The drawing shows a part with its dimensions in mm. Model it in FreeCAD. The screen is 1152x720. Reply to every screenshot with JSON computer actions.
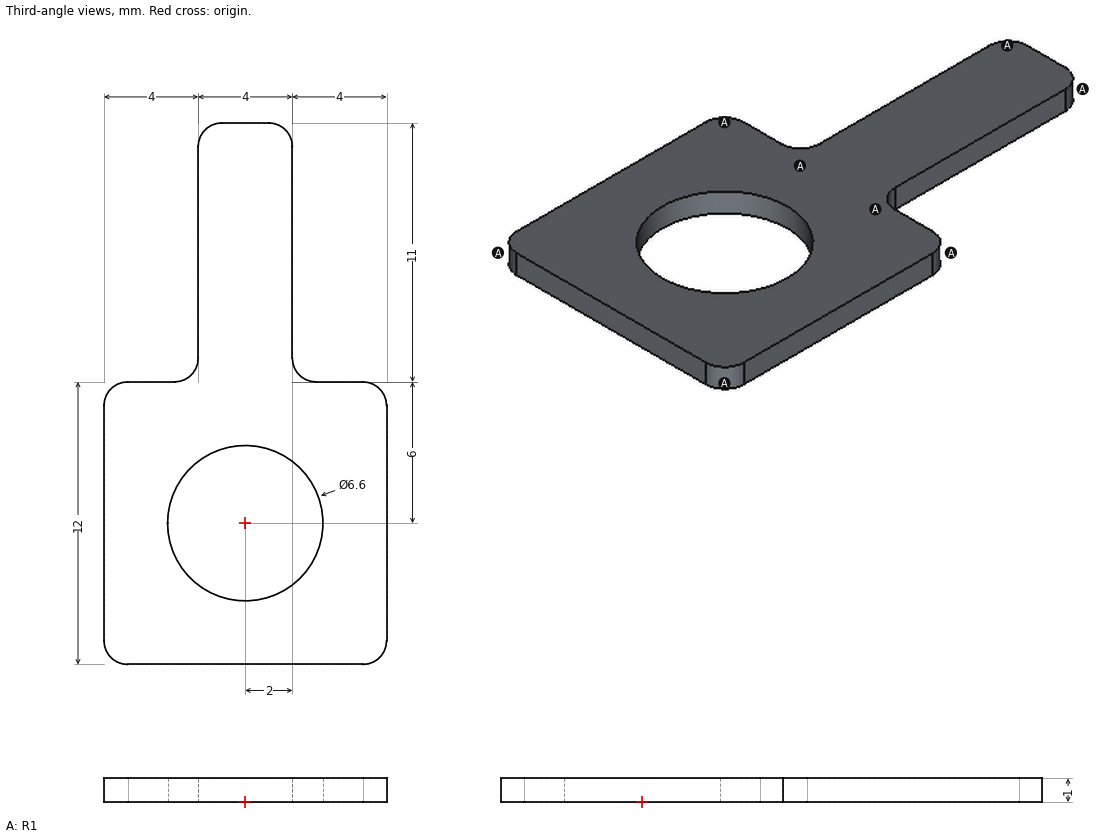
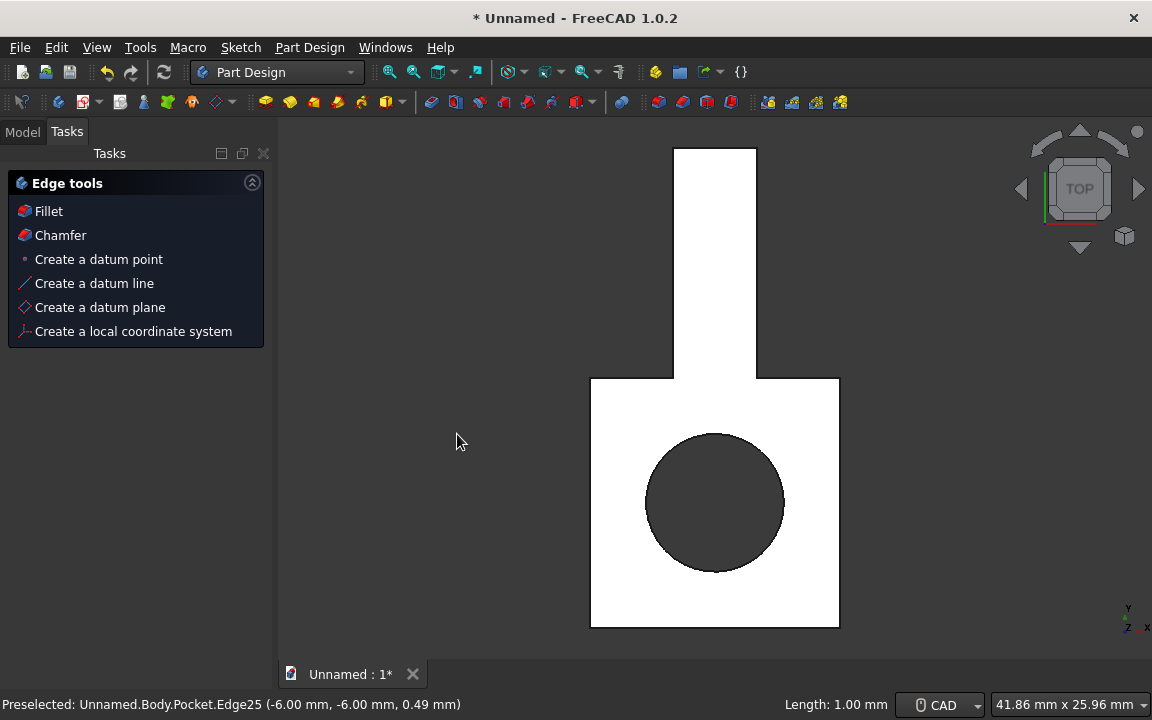
{"action": "scroll", "coordinate": [590, 627], "scroll_direction": "up", "scroll_amount": 4}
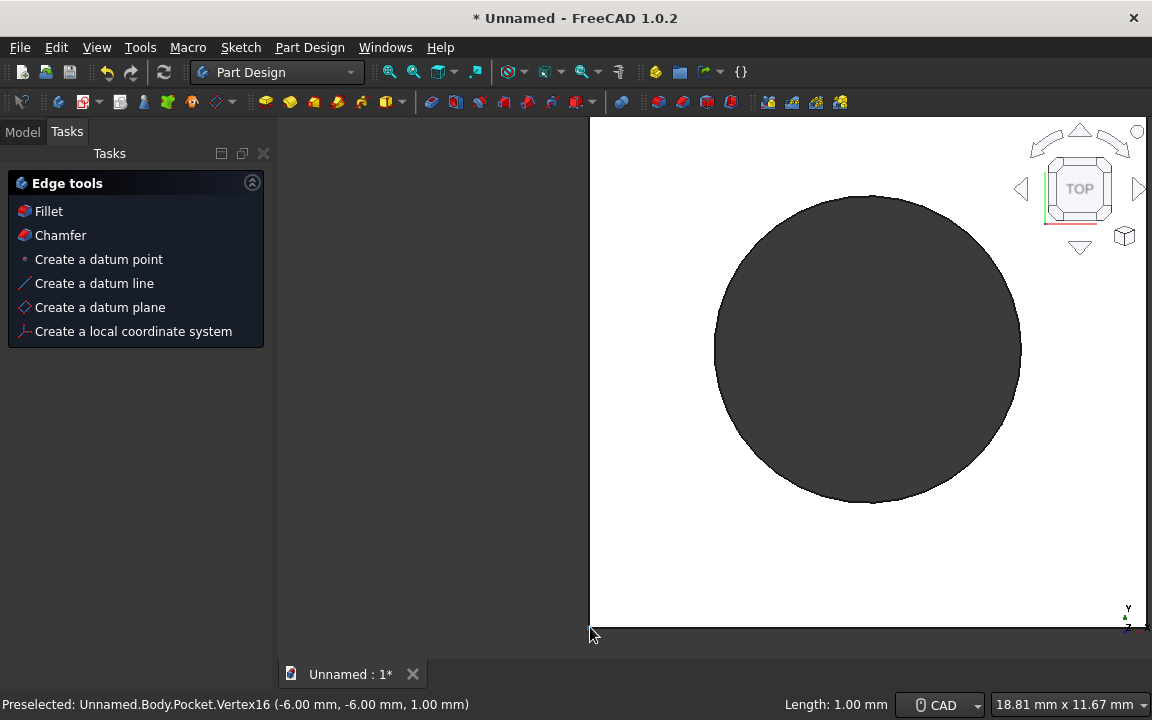
{"action": "key", "text": "v f"}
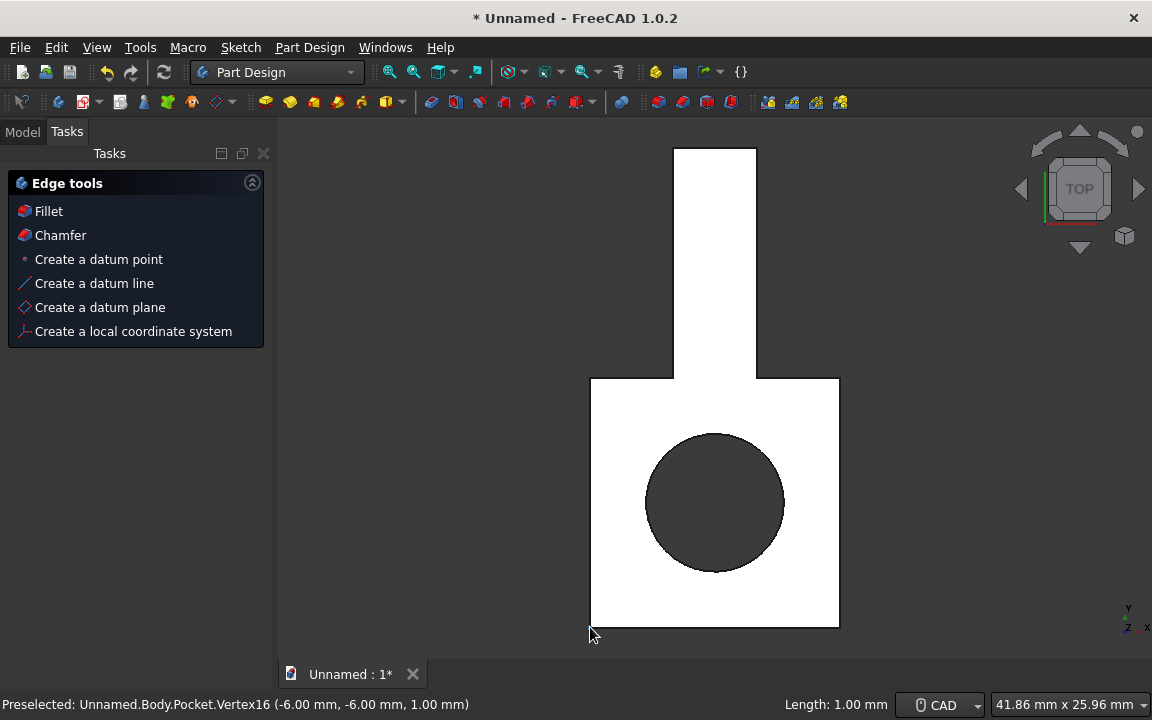
{"action": "key", "text": "1"}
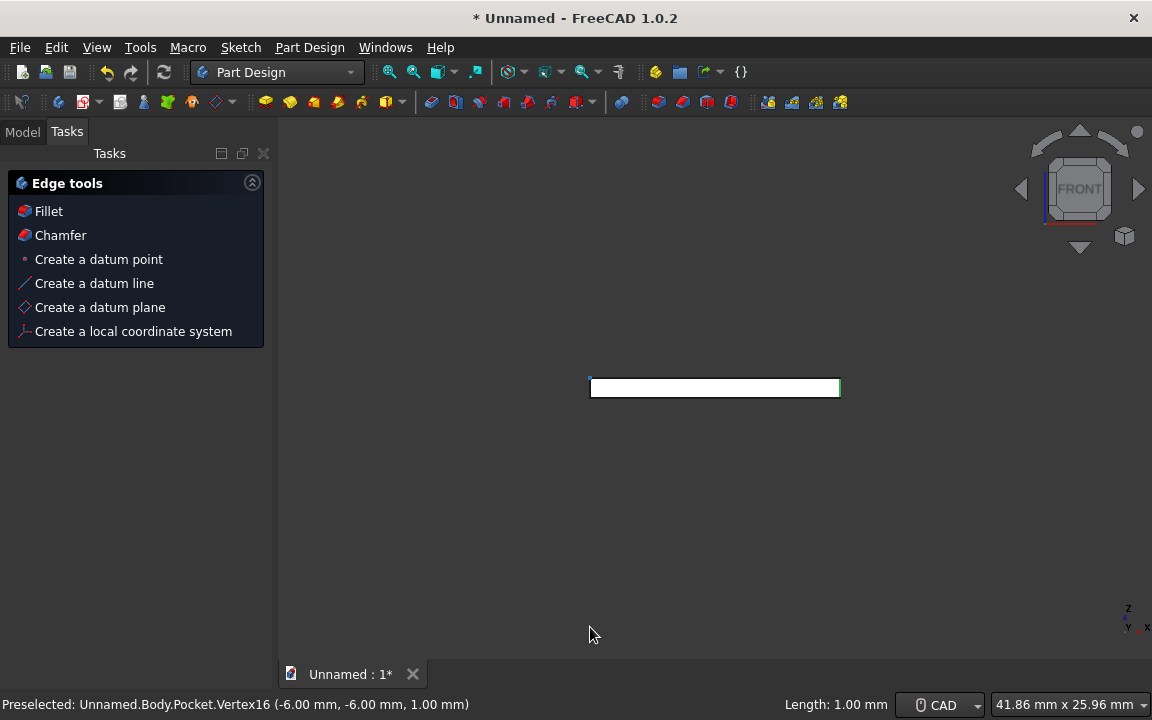
{"action": "left_click", "coordinate": [390, 72]}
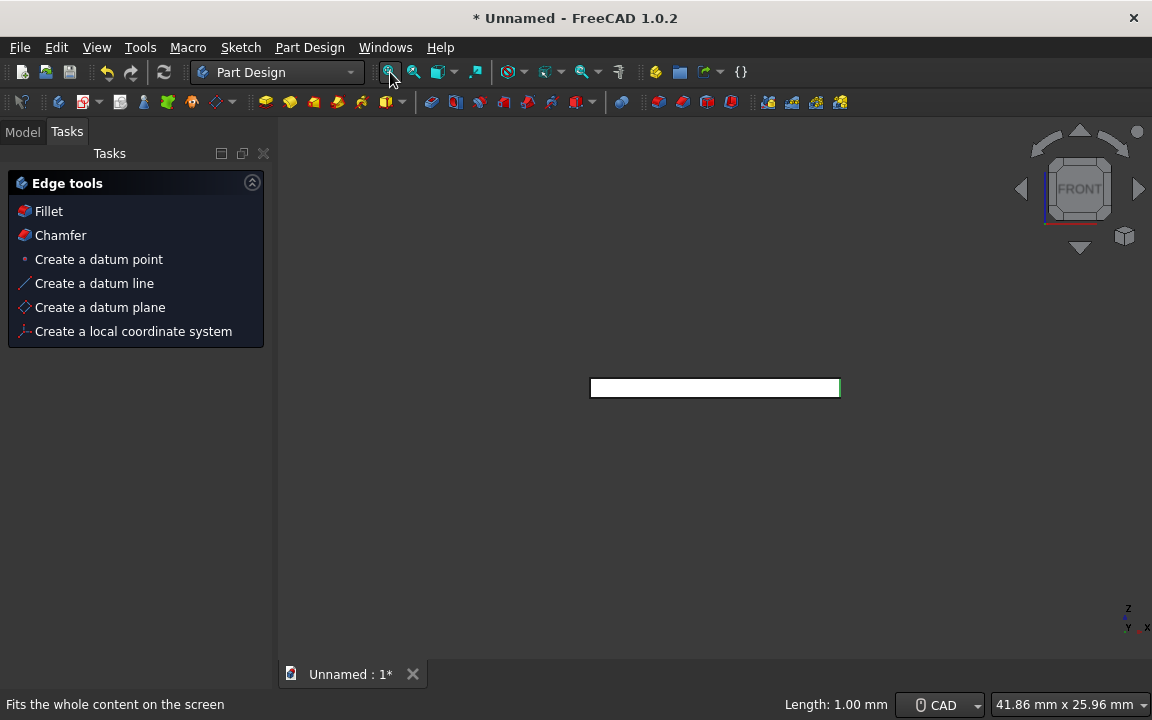
{"action": "left_click", "coordinate": [590, 387], "text": "ctrl"}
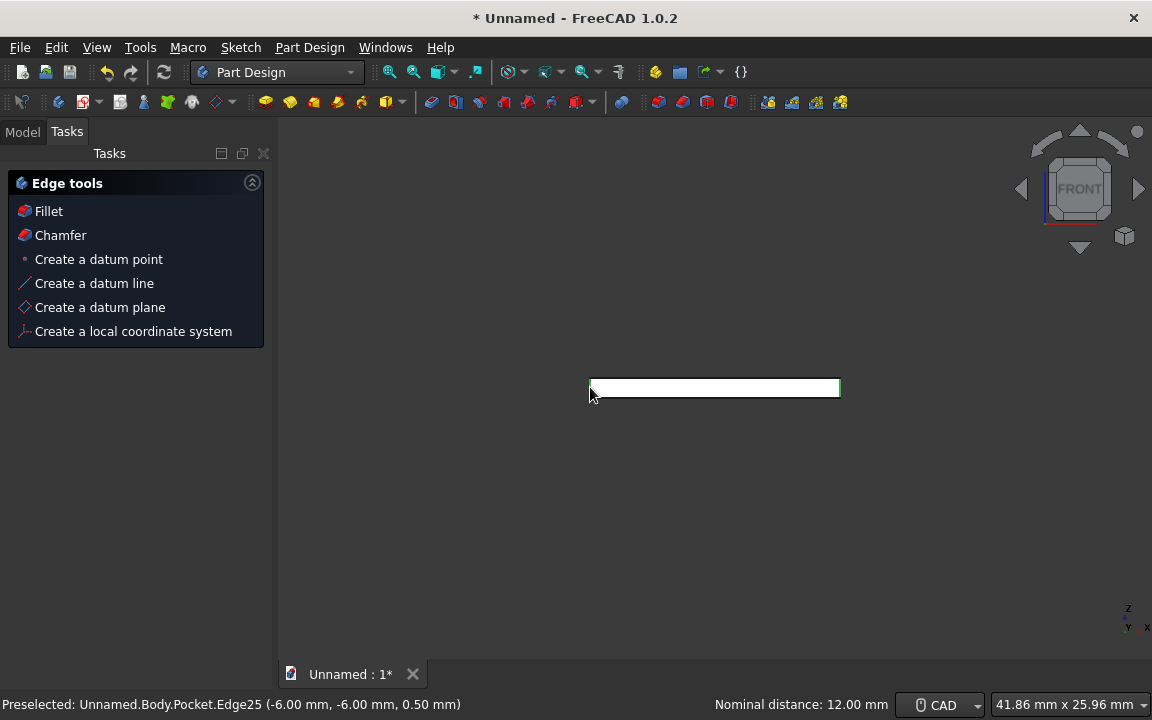
{"action": "scroll", "coordinate": [590, 387], "scroll_direction": "up", "scroll_amount": 4}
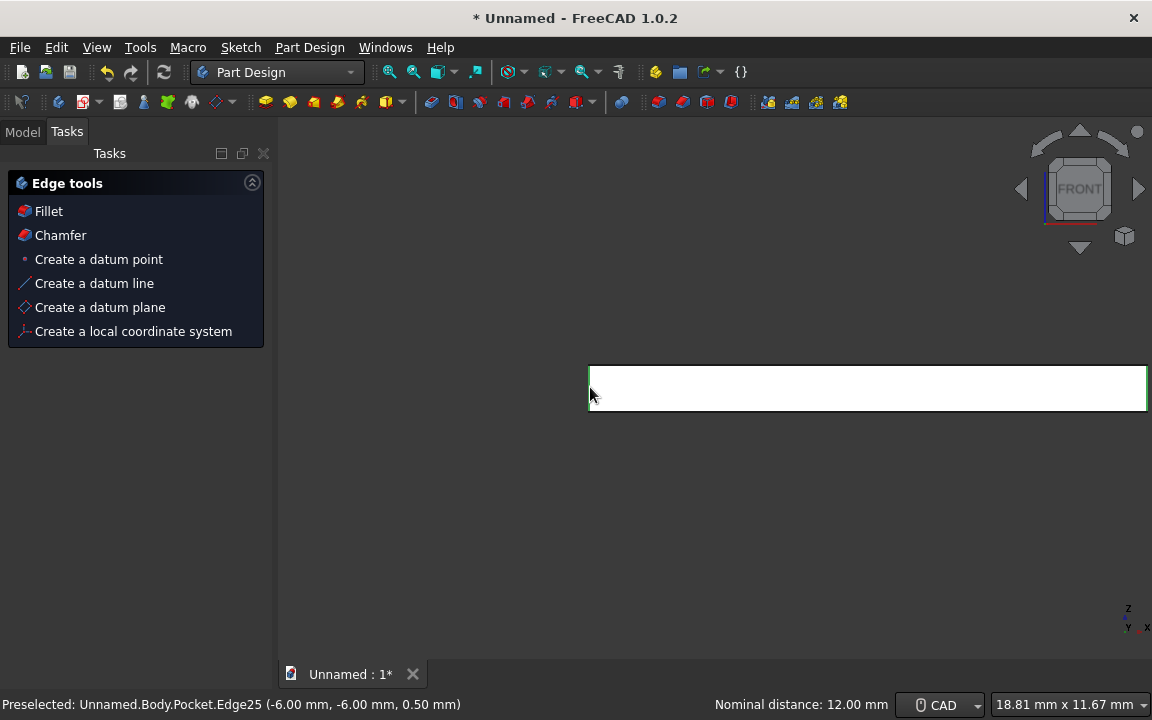
{"action": "key", "text": "v f"}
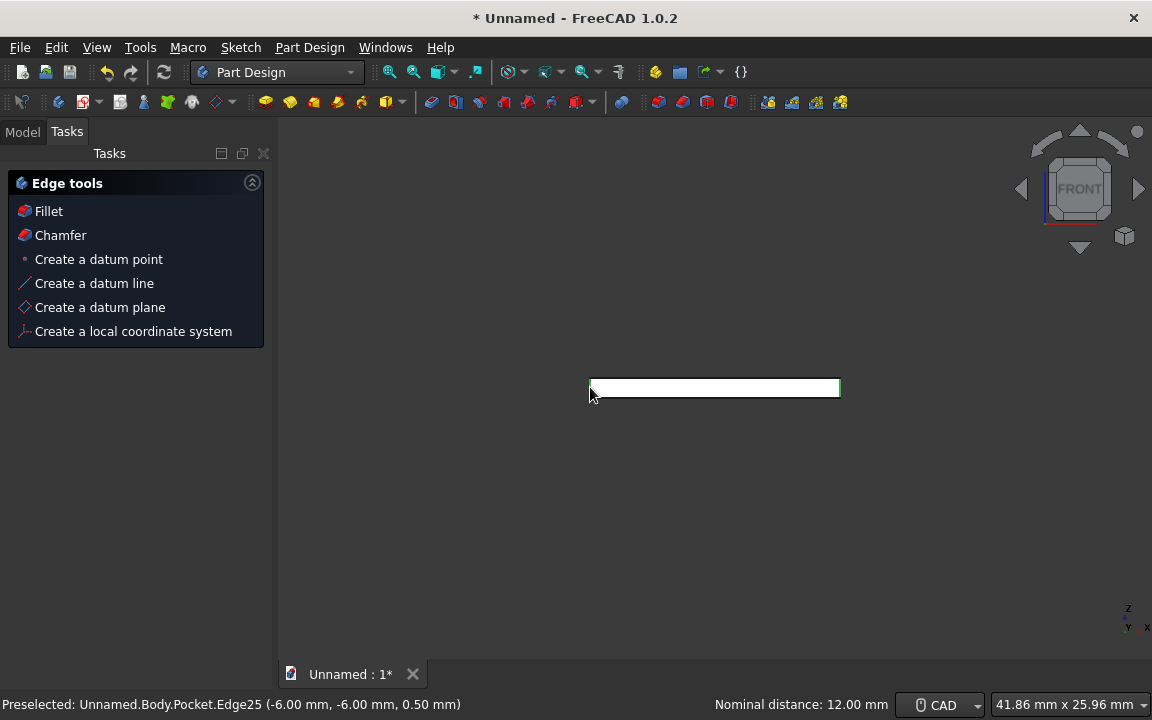
{"action": "key", "text": "3"}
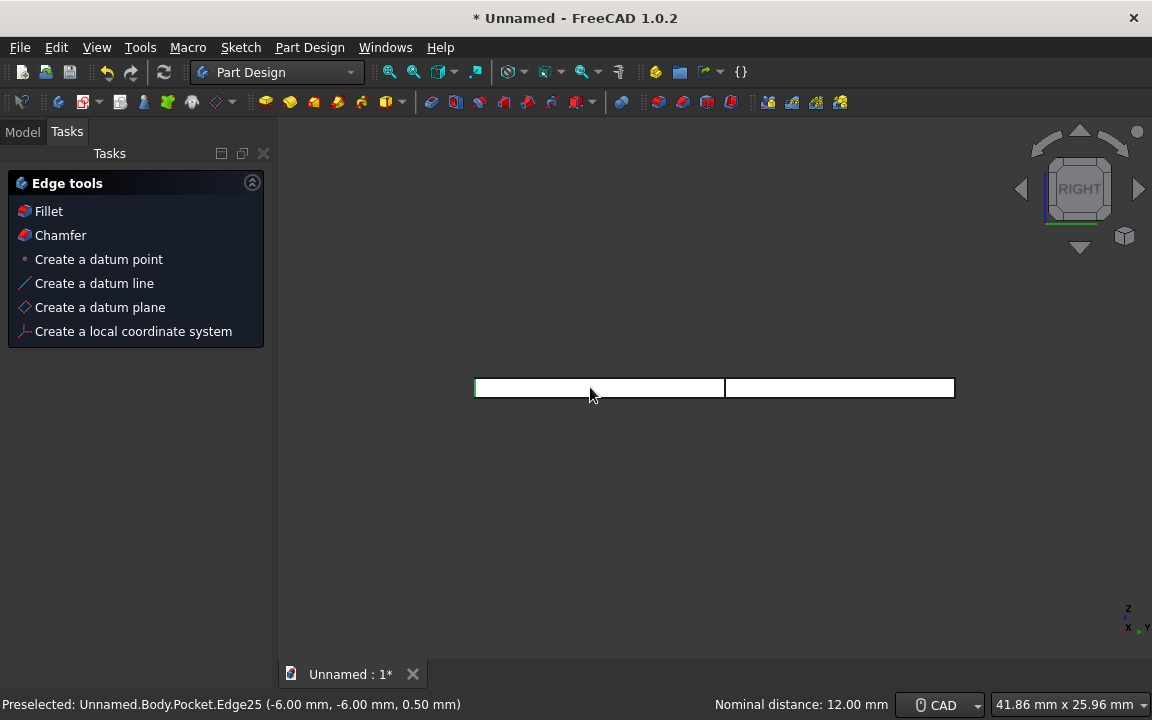
{"action": "left_click", "coordinate": [955, 387], "text": "ctrl"}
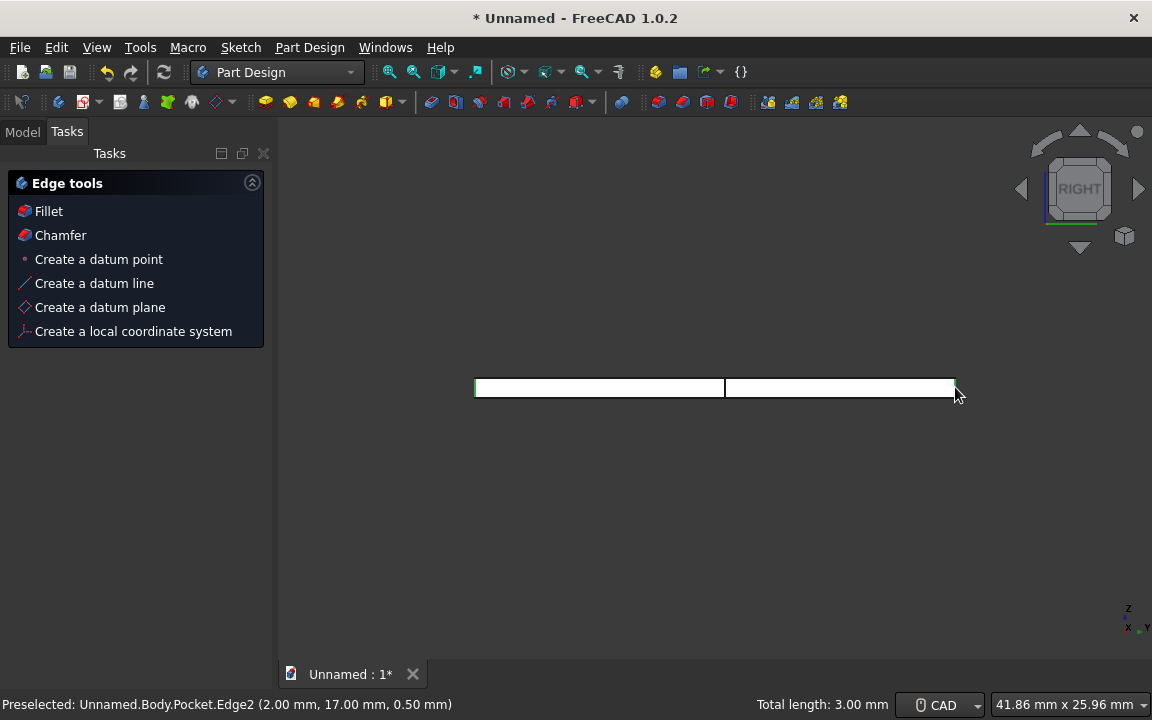
{"action": "left_click", "coordinate": [725, 387], "text": "ctrl"}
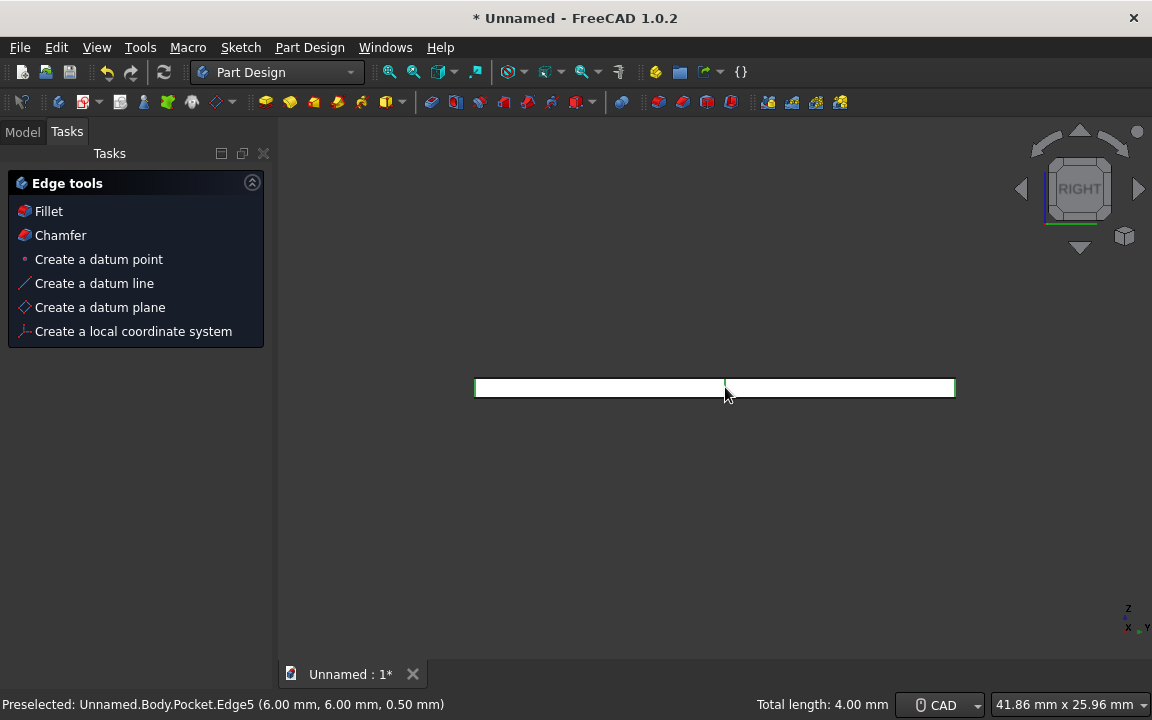
{"action": "scroll", "coordinate": [725, 387], "scroll_direction": "up", "scroll_amount": 4}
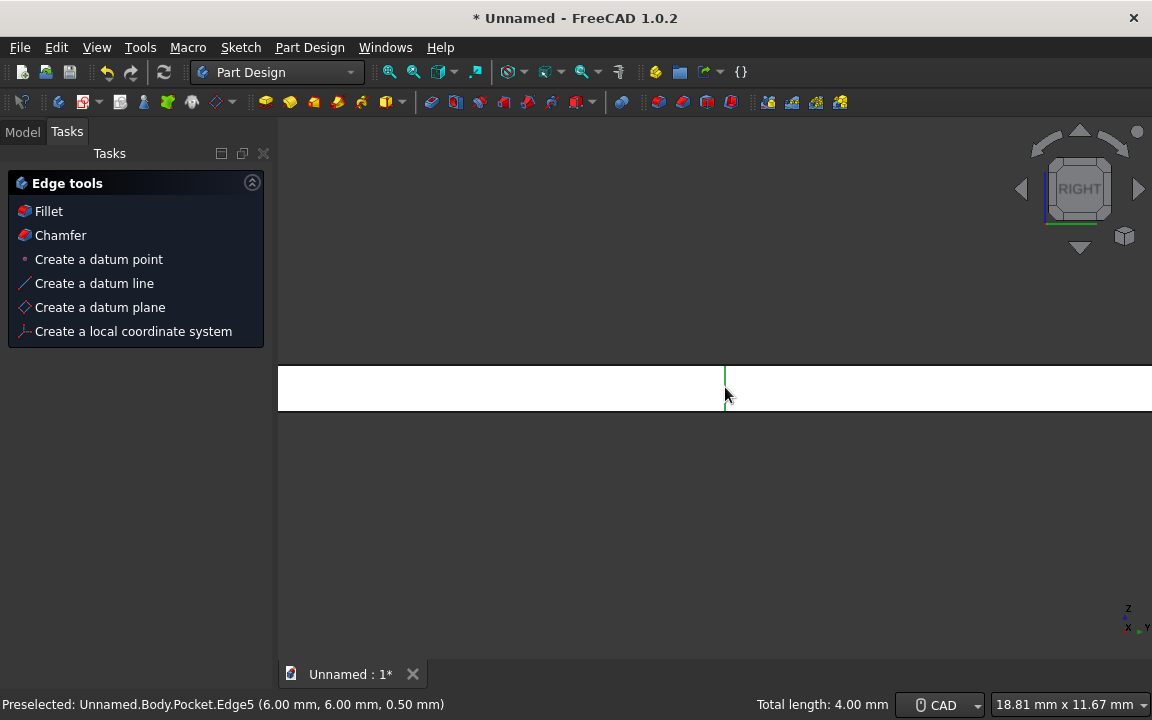
{"action": "key", "text": "v f"}